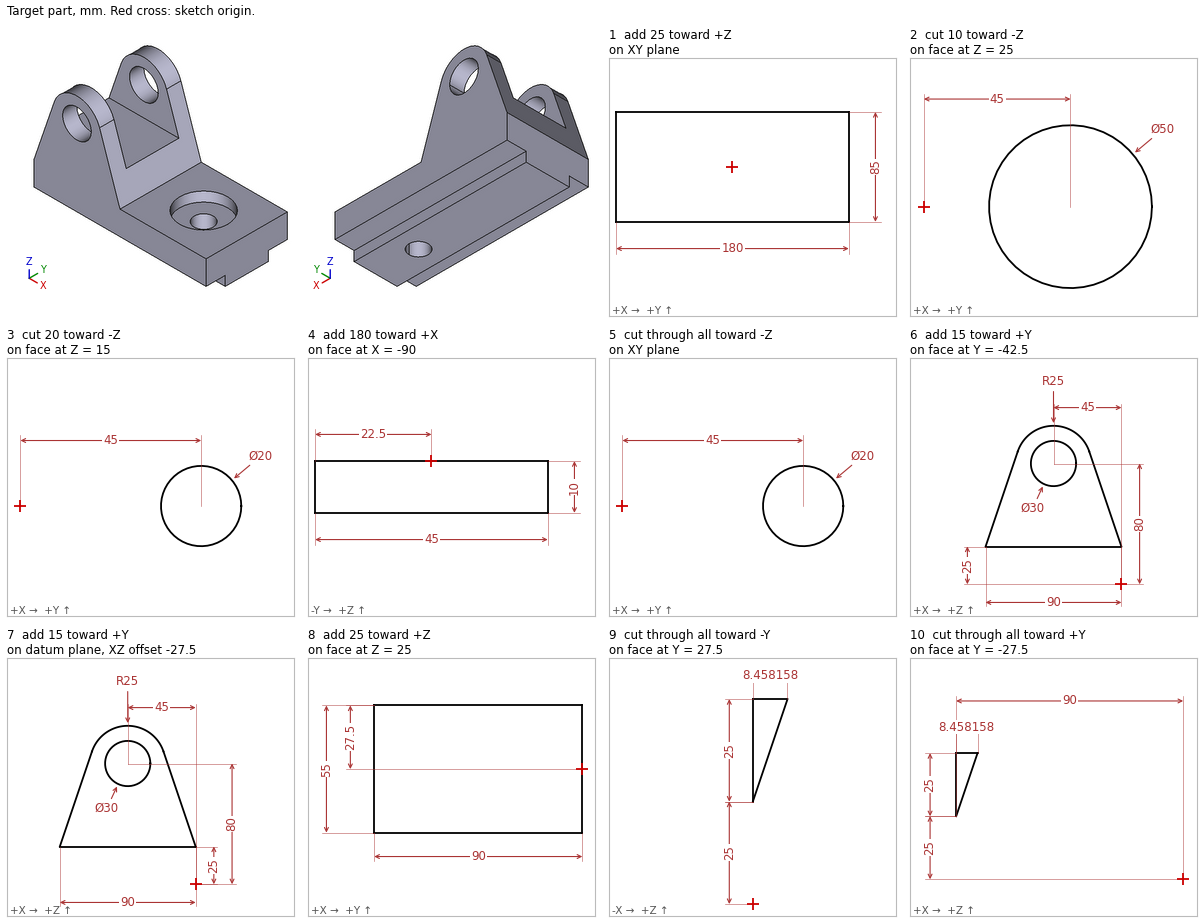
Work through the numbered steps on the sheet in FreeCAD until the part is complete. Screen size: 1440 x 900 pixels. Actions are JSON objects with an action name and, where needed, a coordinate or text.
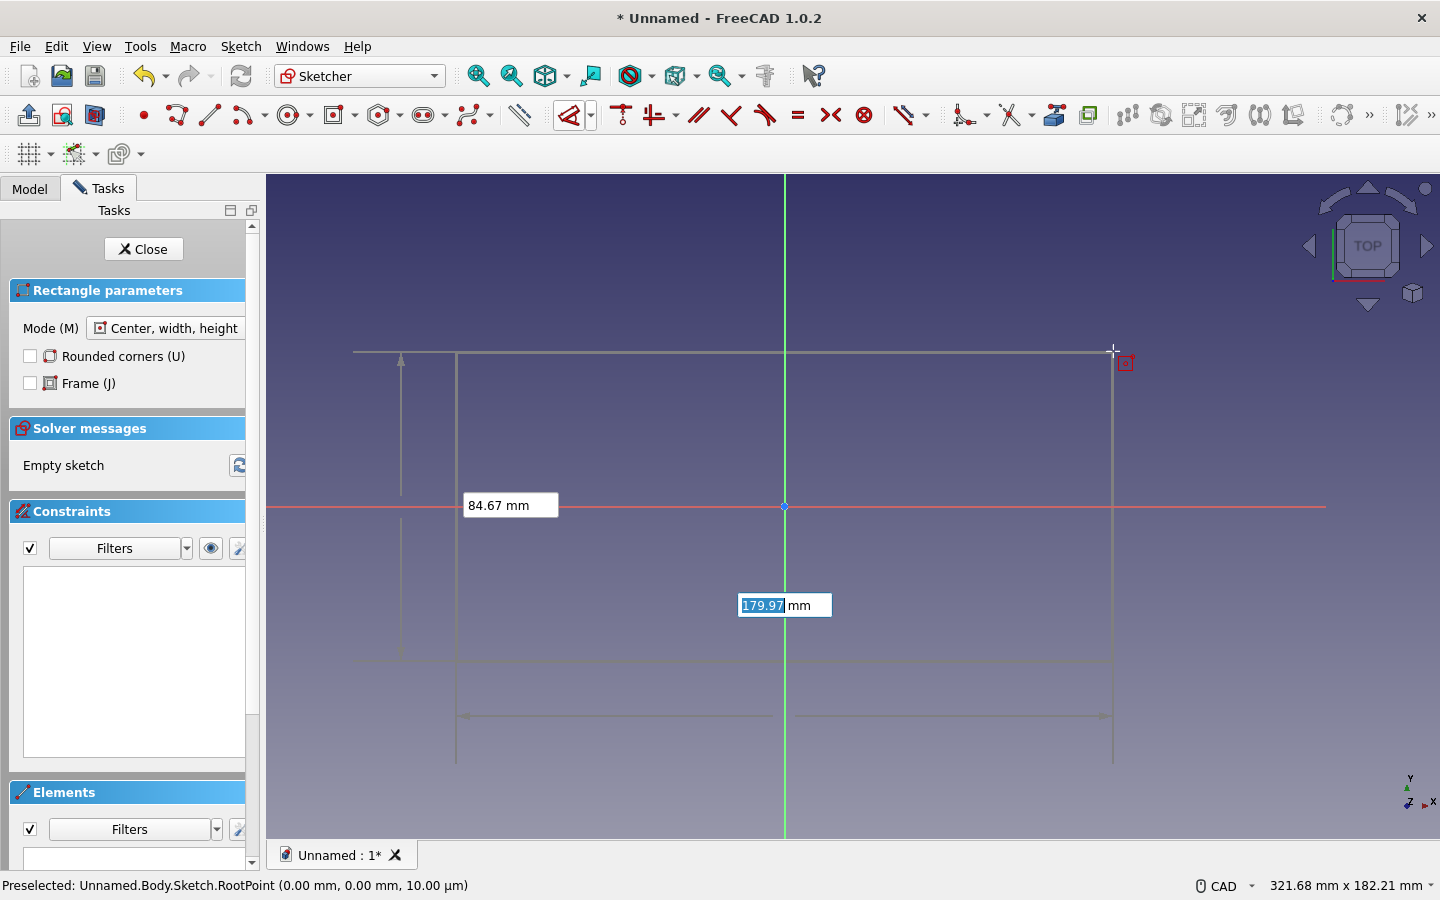
{"action": "type", "text": "180"}
{"action": "key", "text": "Tab"}
{"action": "type", "text": "85"}
{"action": "key", "text": "Return"}
{"action": "key", "text": "Escape"}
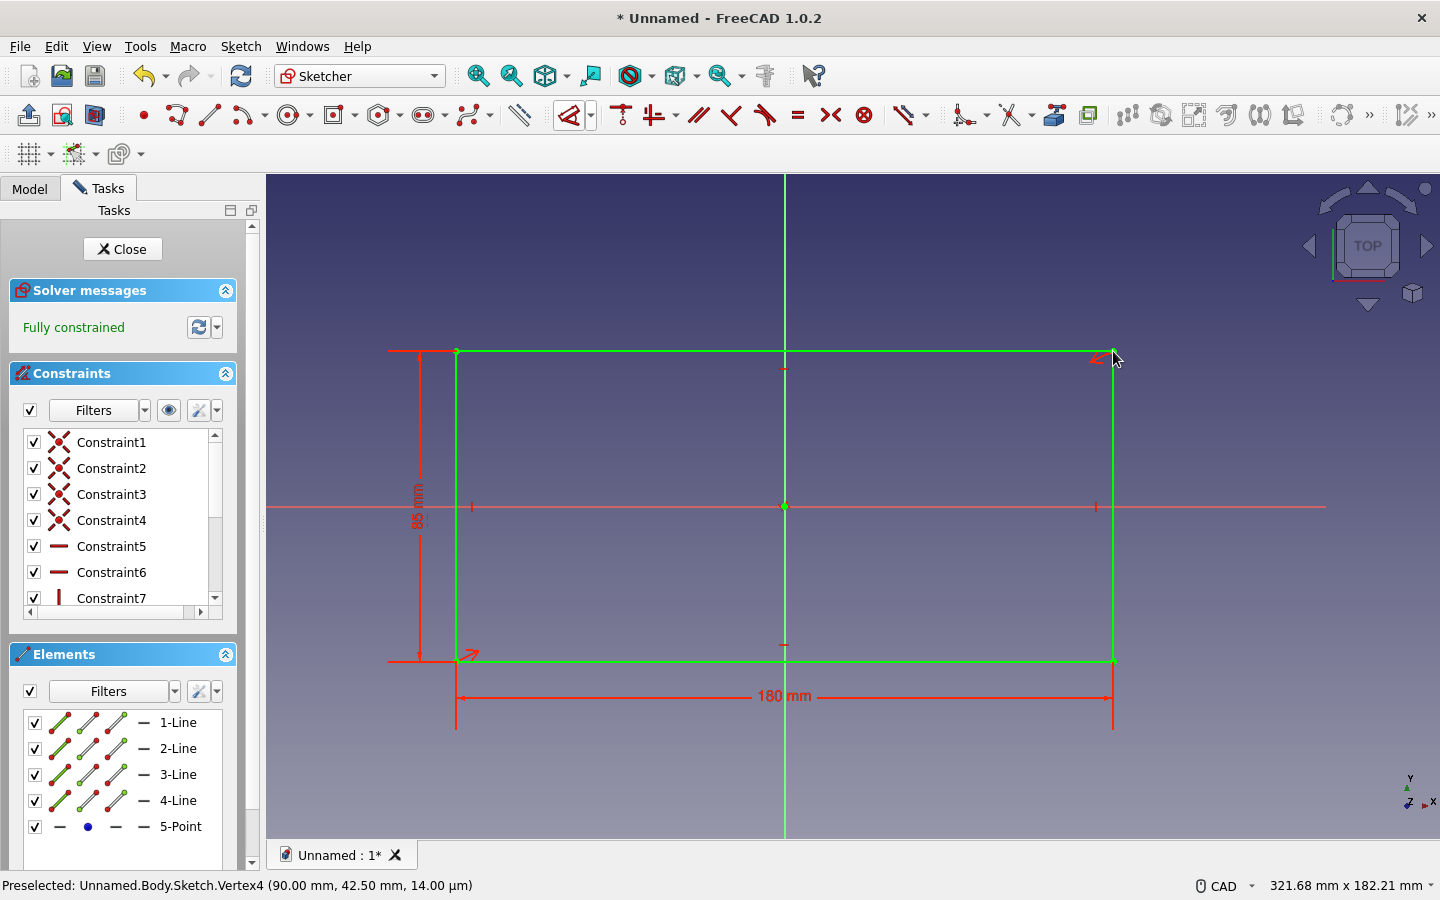
{"action": "left_click", "coordinate": [123, 249]}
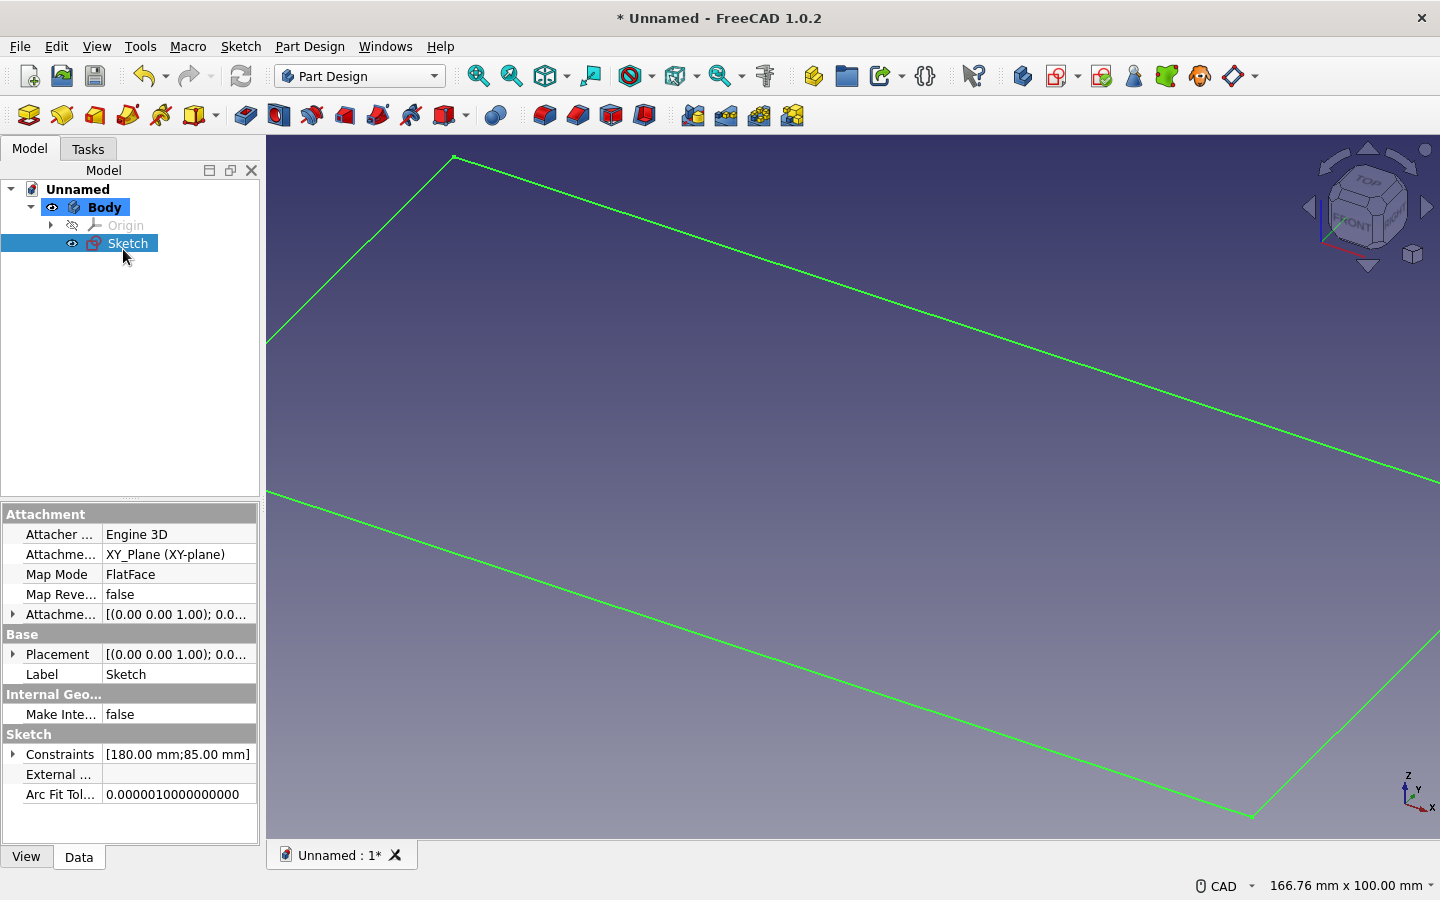
{"action": "left_click", "coordinate": [29, 116]}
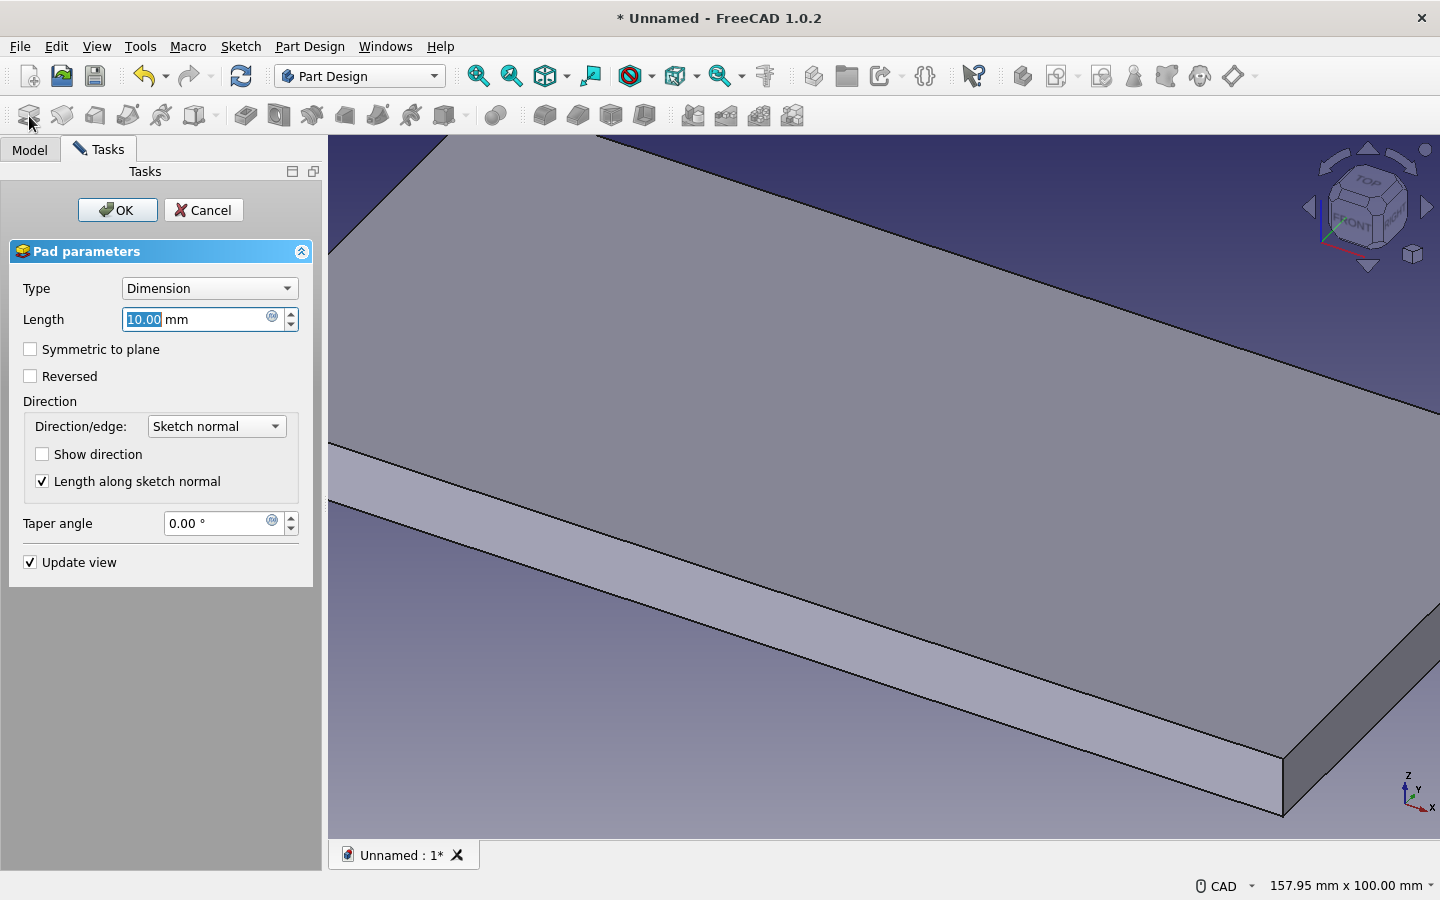
{"action": "type", "text": "25"}
{"action": "key", "text": "Tab"}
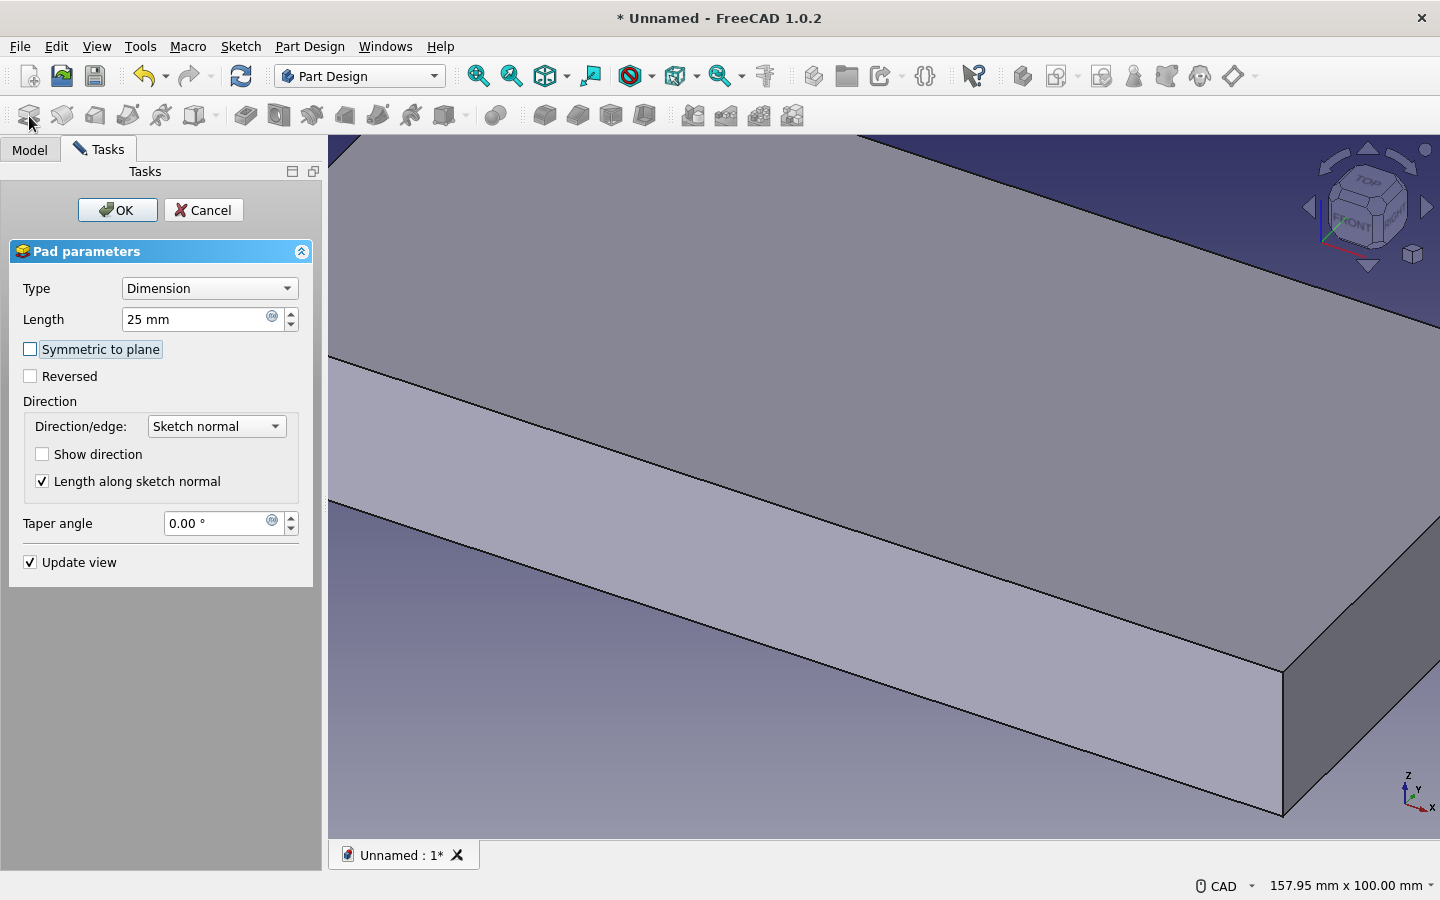
{"action": "left_click", "coordinate": [118, 210]}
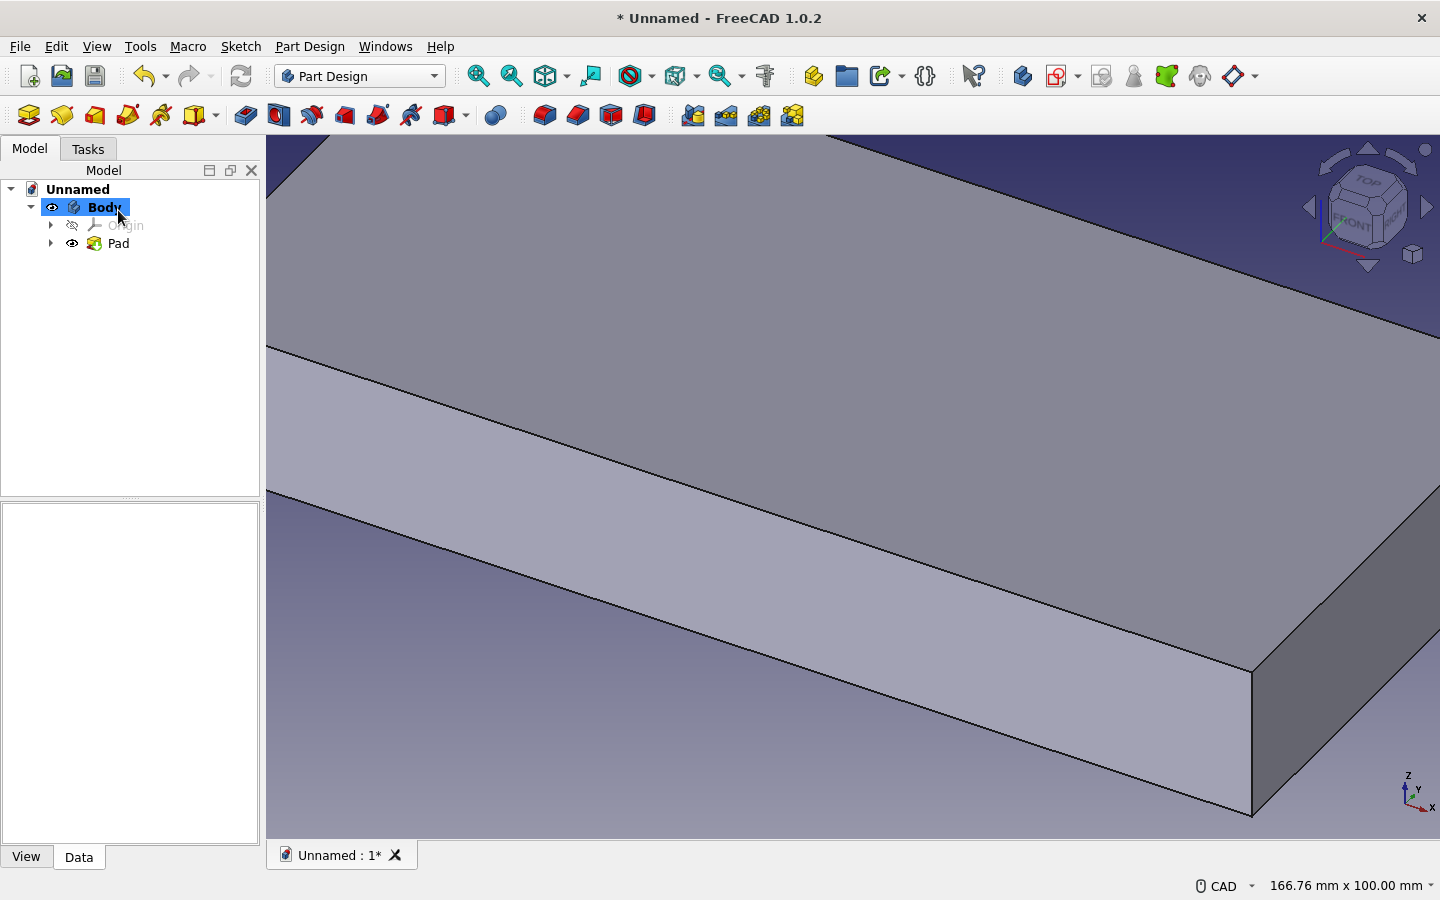
{"action": "left_click", "coordinate": [479, 76]}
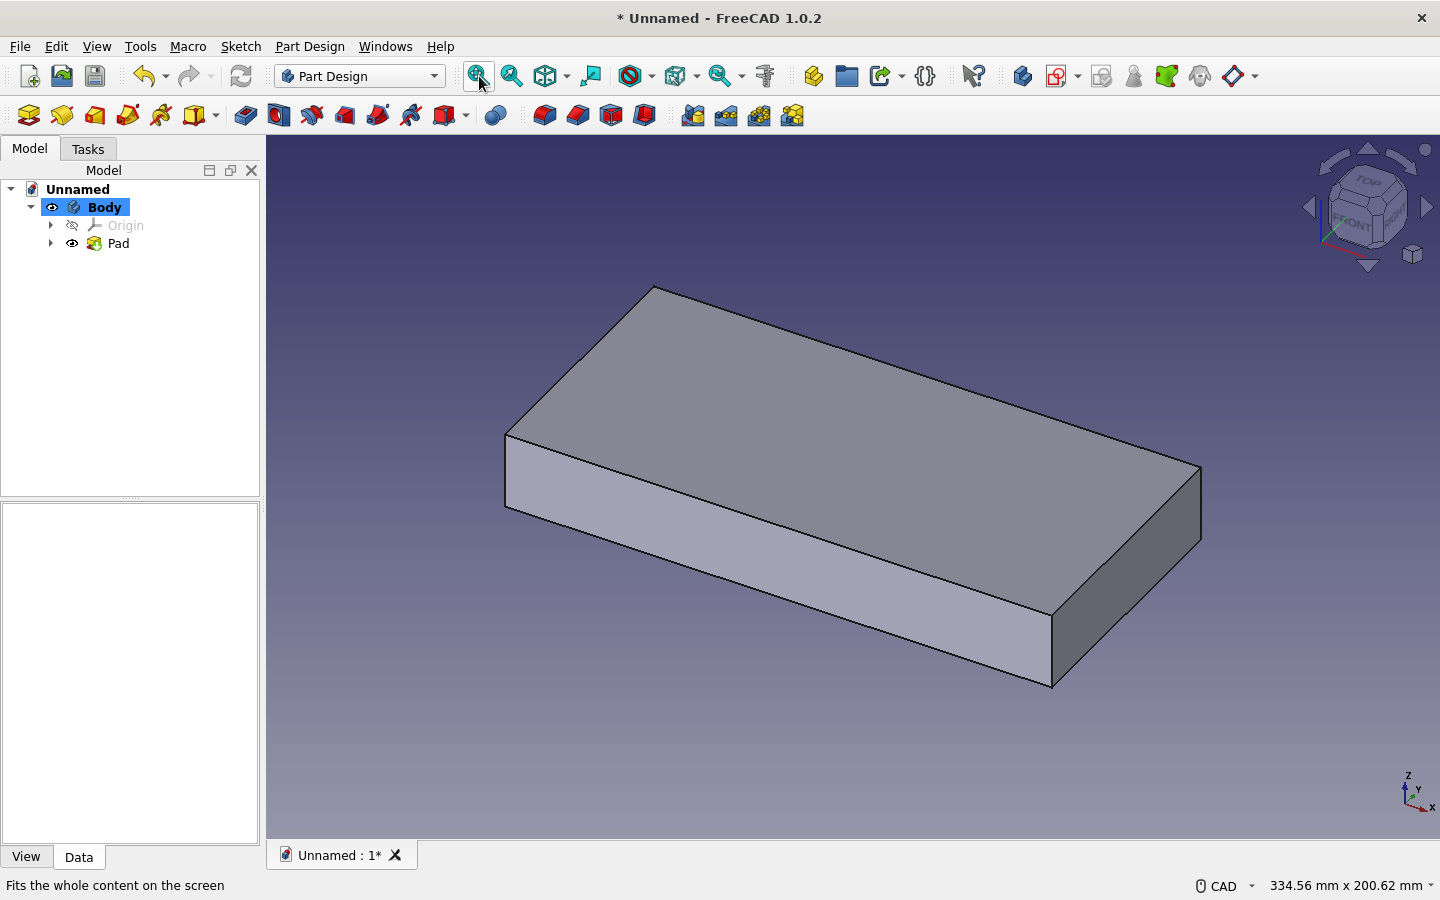
{"action": "left_click", "coordinate": [931, 476]}